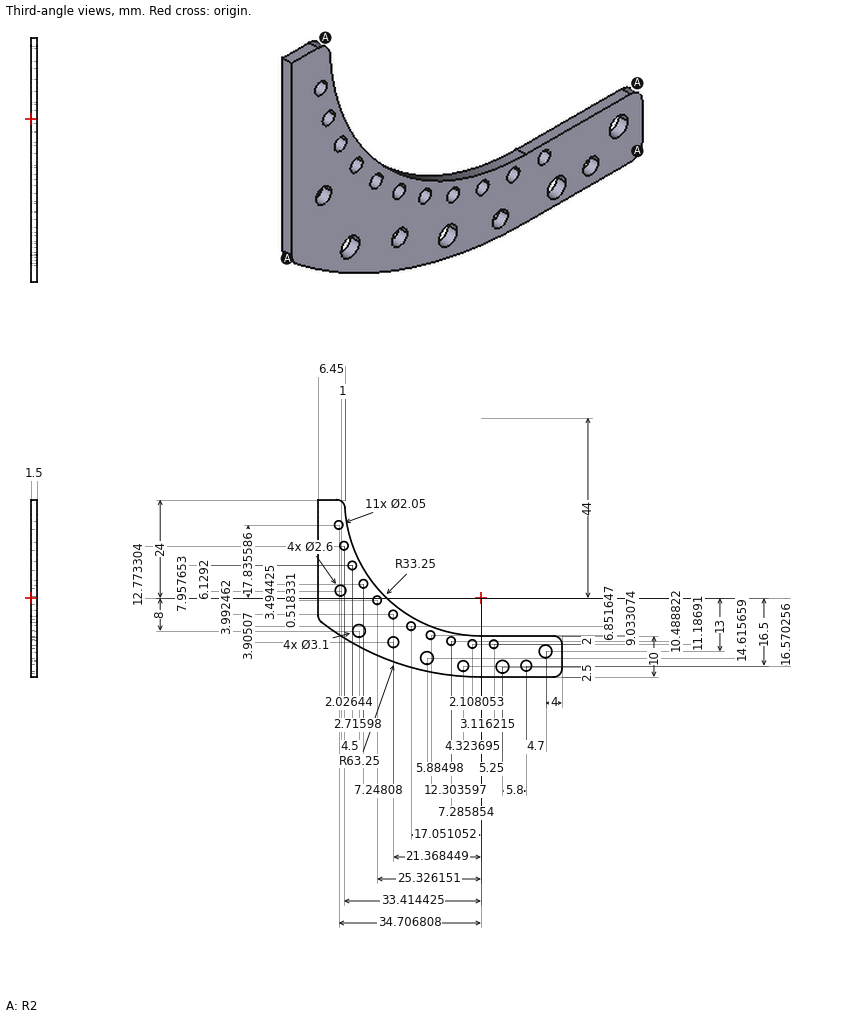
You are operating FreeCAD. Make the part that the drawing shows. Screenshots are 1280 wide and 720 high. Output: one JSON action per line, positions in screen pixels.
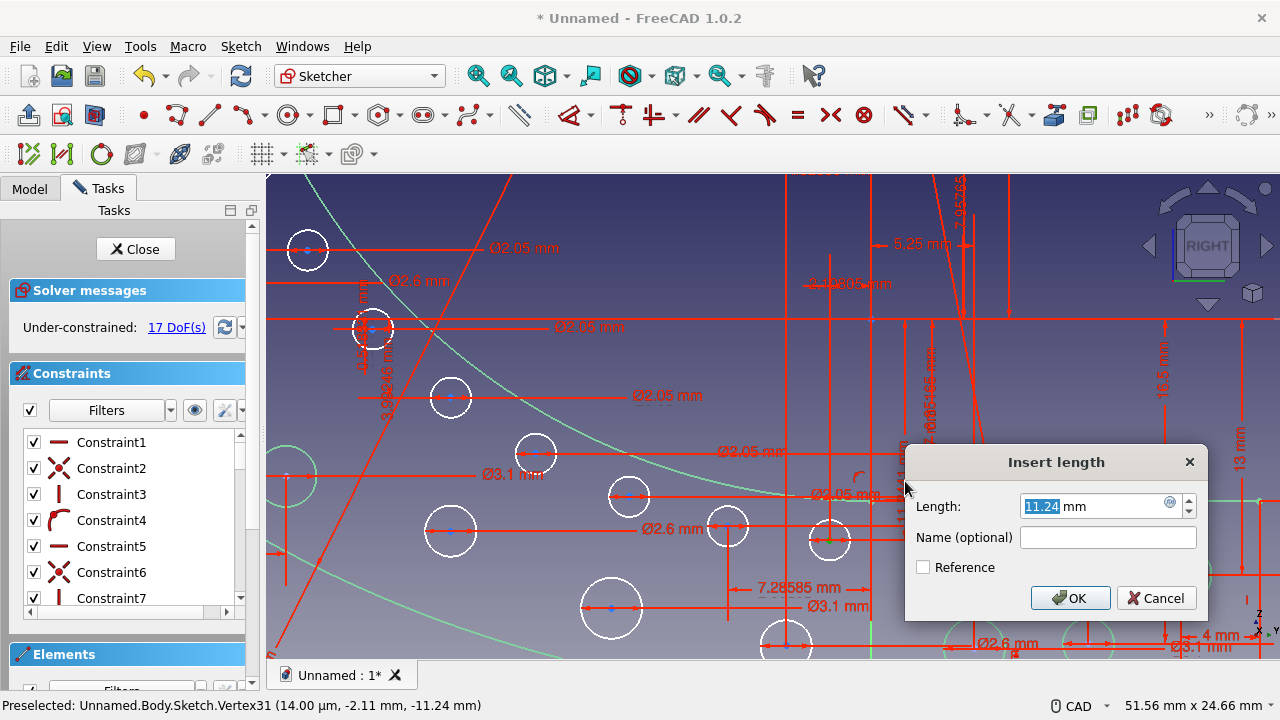
{"action": "type", "text": "11.18691"}
{"action": "key", "text": "Return"}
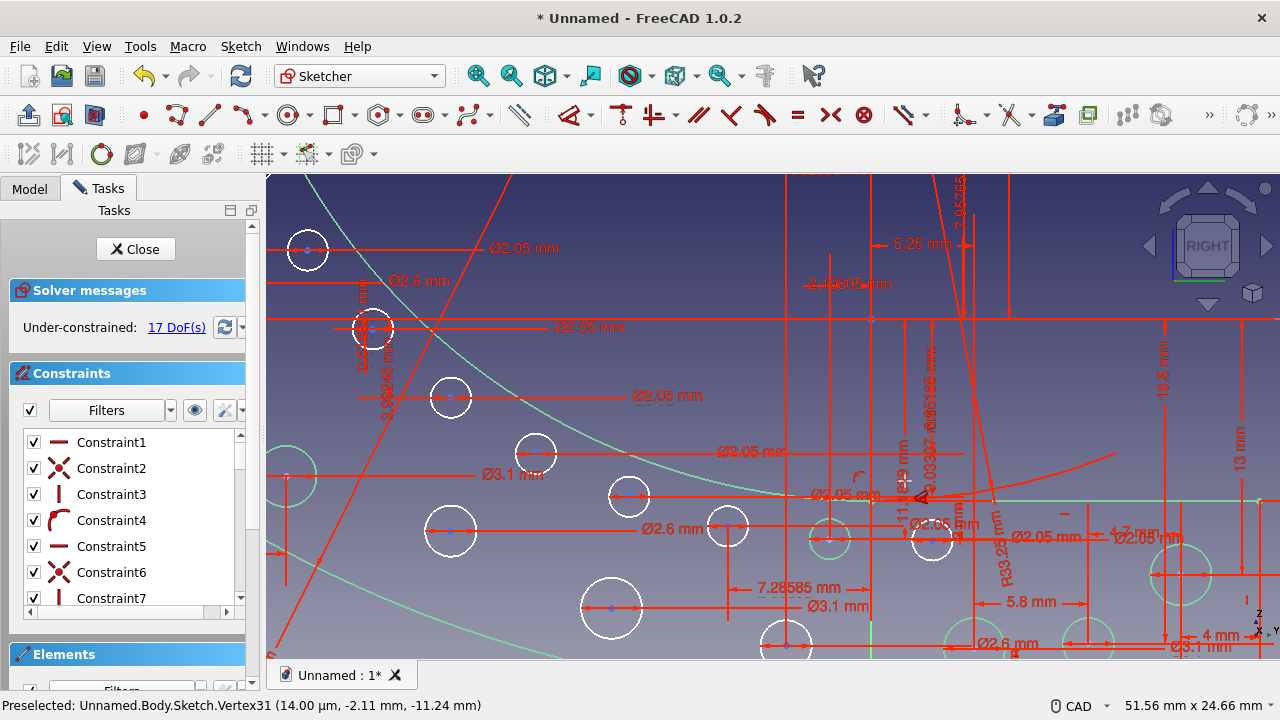
{"action": "left_click", "coordinate": [932, 540]}
{"action": "left_click", "coordinate": [902, 574]}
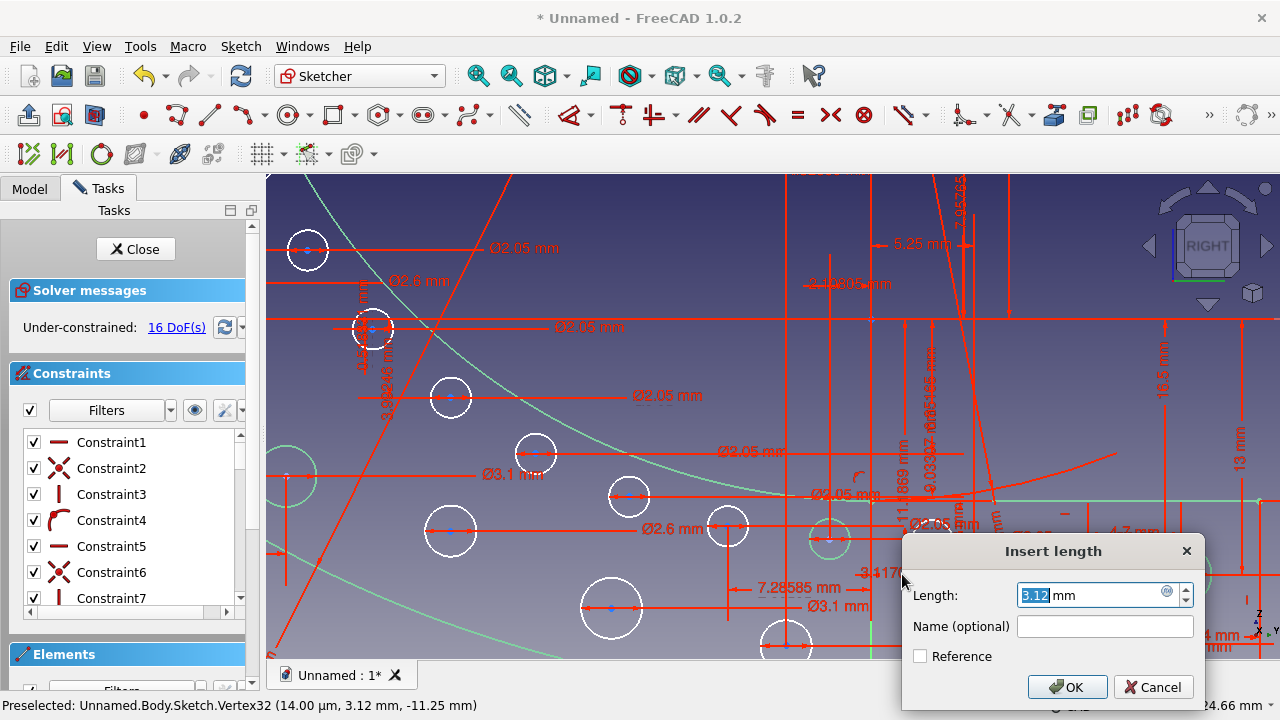
{"action": "type", "text": "3.116215"}
{"action": "key", "text": "Return"}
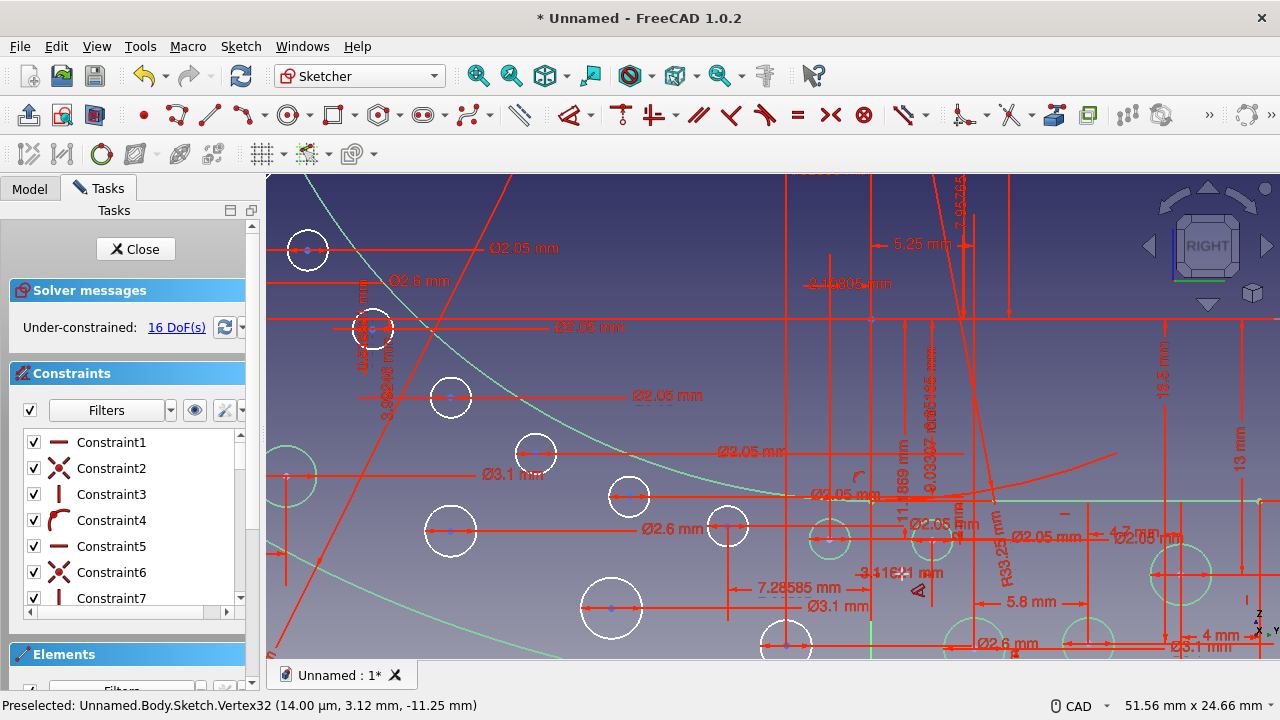
{"action": "scroll", "coordinate": [722, 500], "scroll_direction": "down", "scroll_amount": 5}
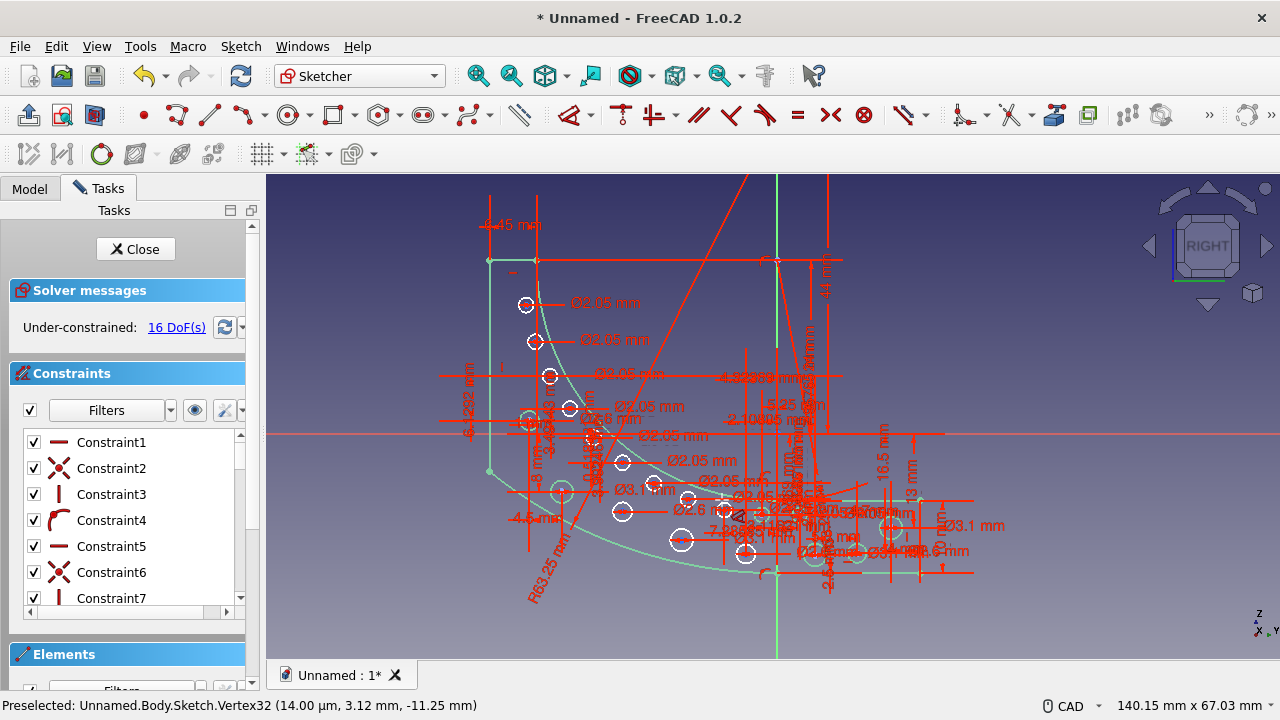
{"action": "scroll", "coordinate": [535, 342], "scroll_direction": "up", "scroll_amount": 5}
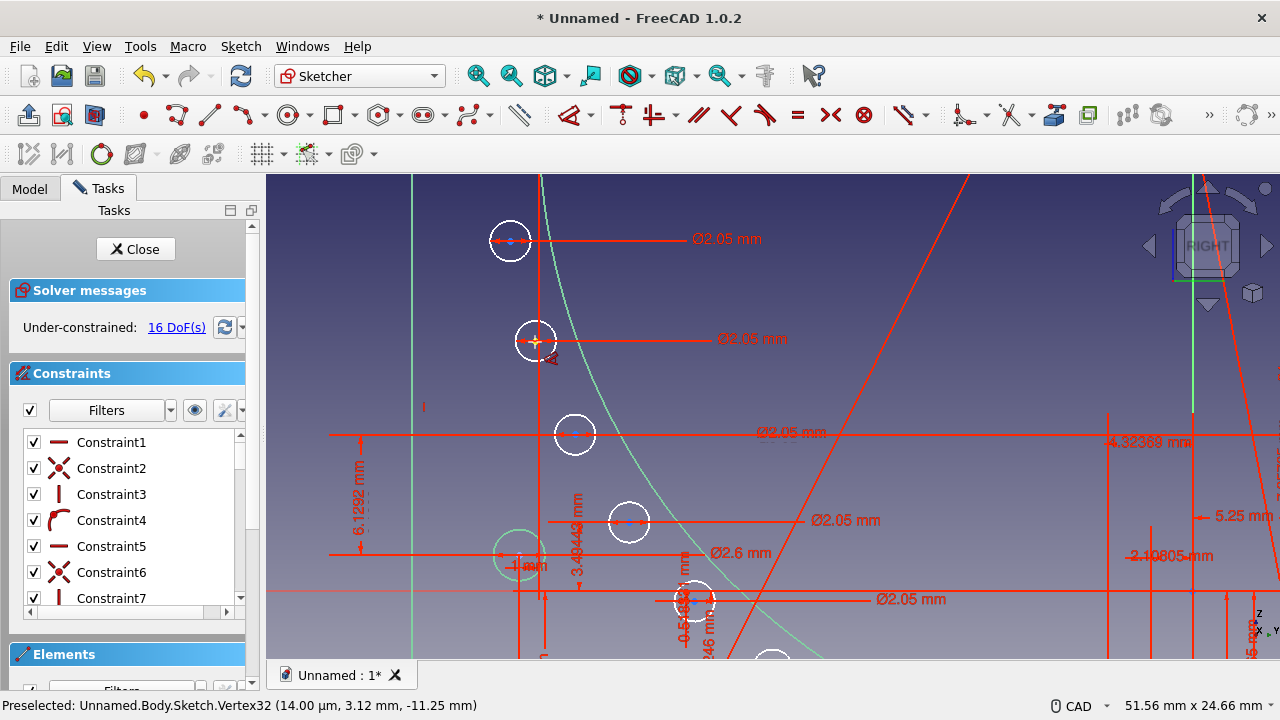
{"action": "left_click", "coordinate": [536, 341]}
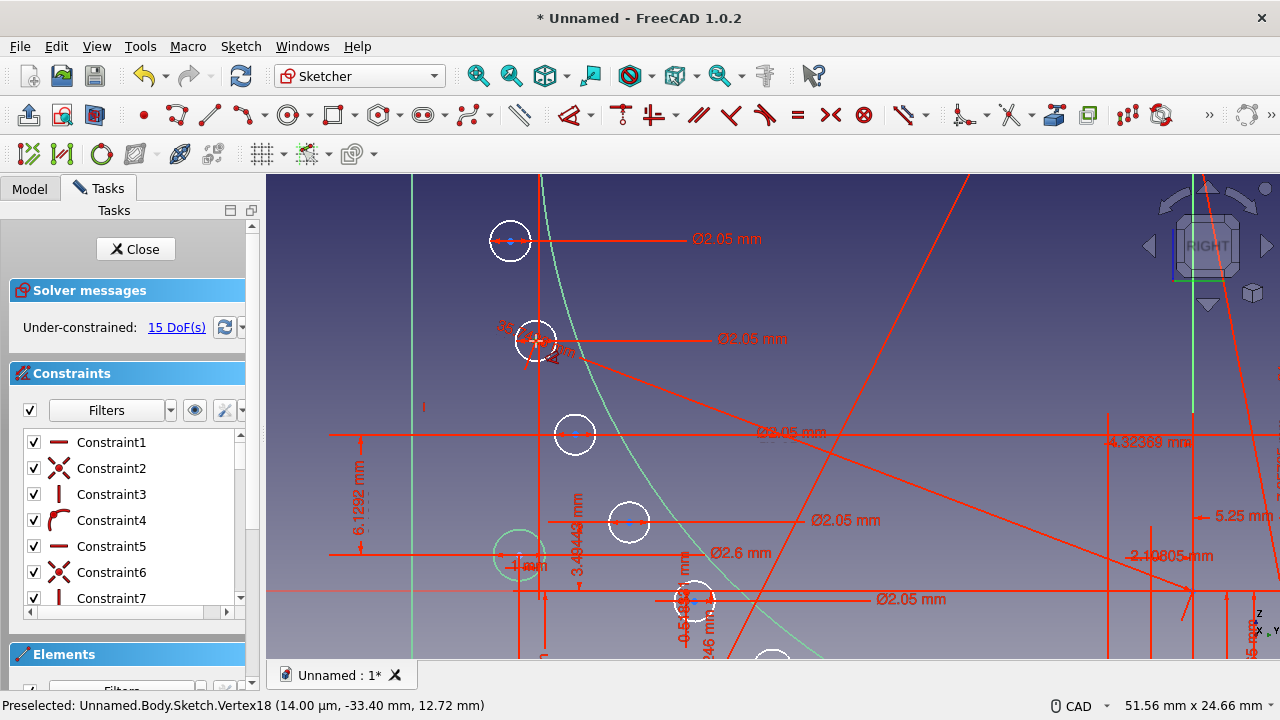
{"action": "left_click", "coordinate": [575, 435]}
{"action": "left_click", "coordinate": [546, 307]}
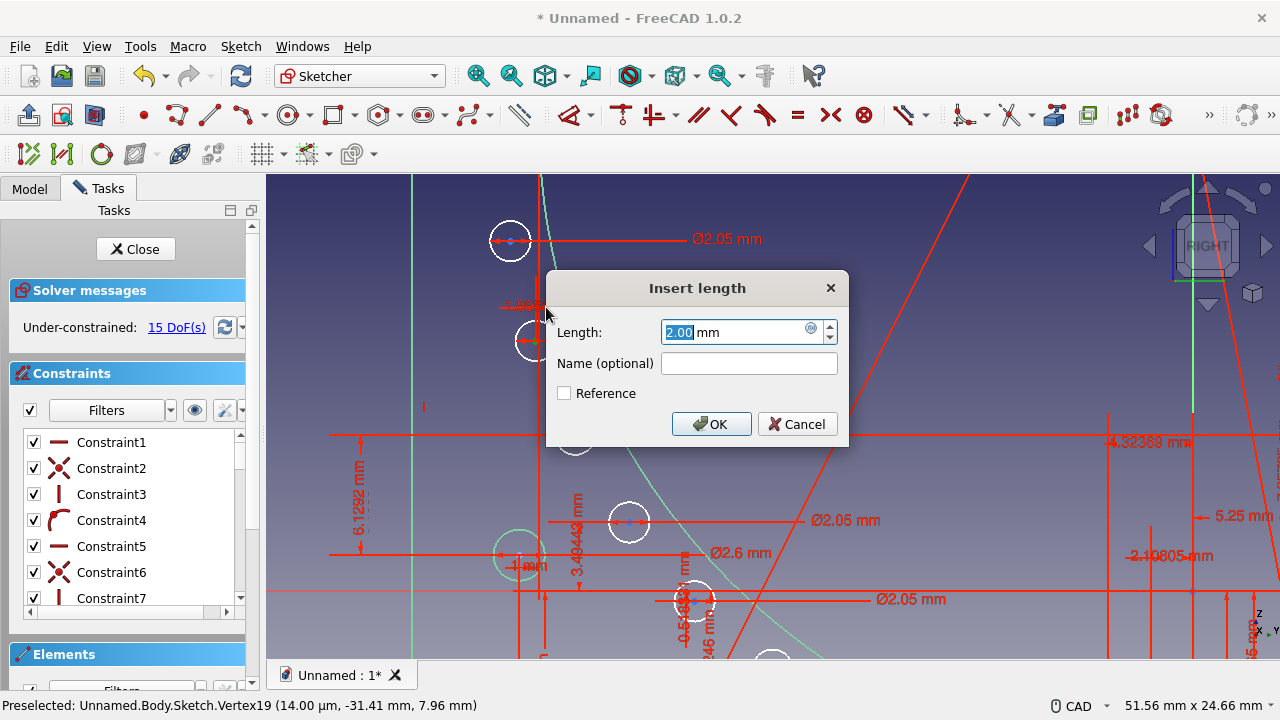
{"action": "type", "text": "2.02644"}
{"action": "key", "text": "Return"}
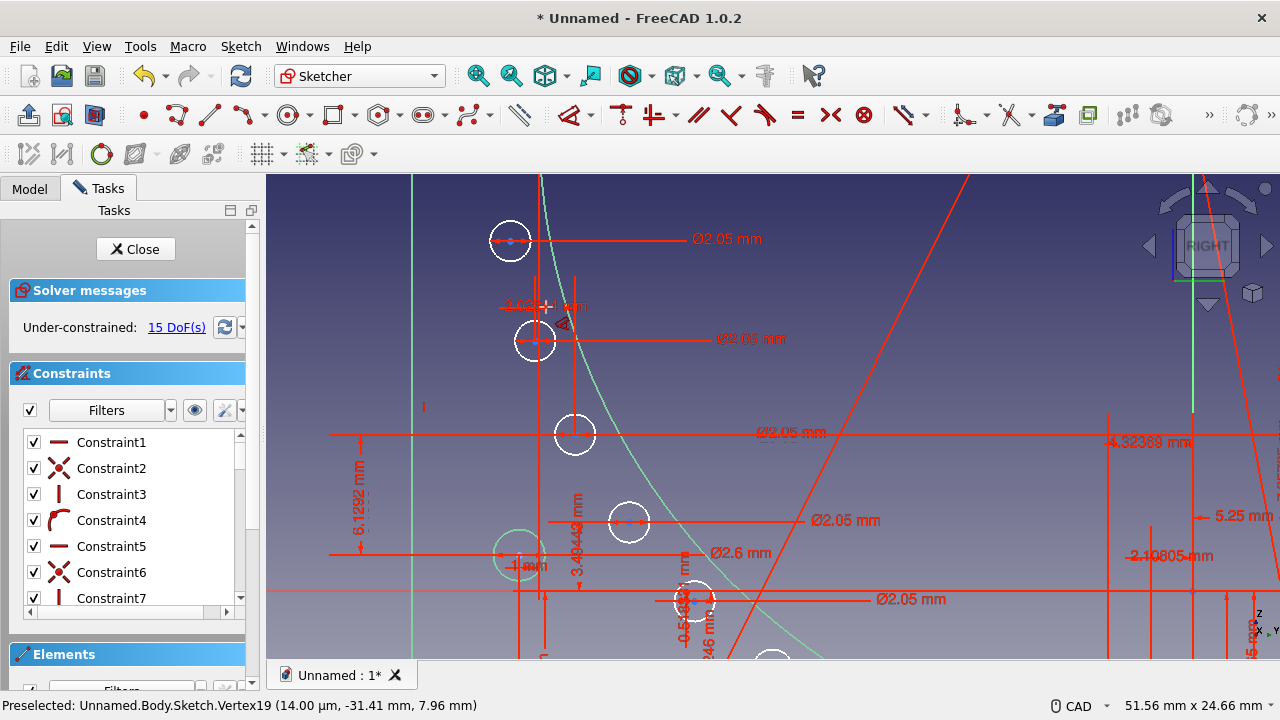
{"action": "left_click", "coordinate": [575, 435]}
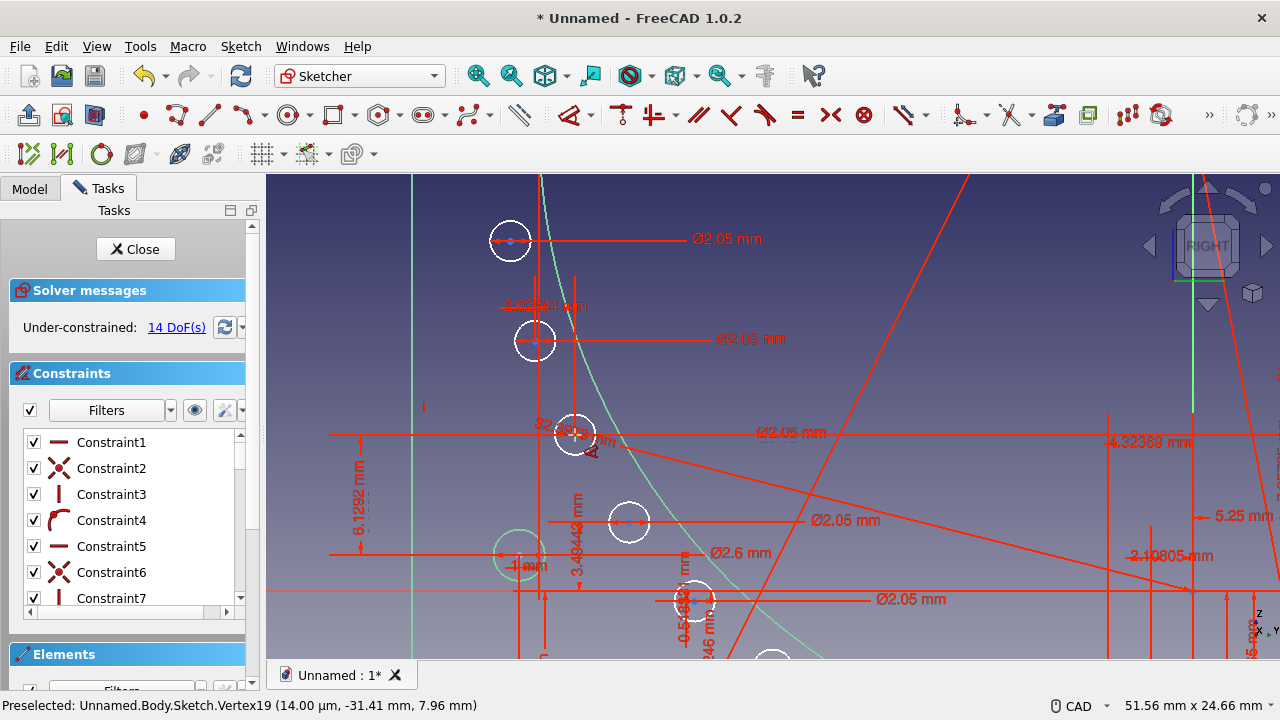
{"action": "left_click", "coordinate": [629, 522]}
{"action": "left_click", "coordinate": [583, 401]}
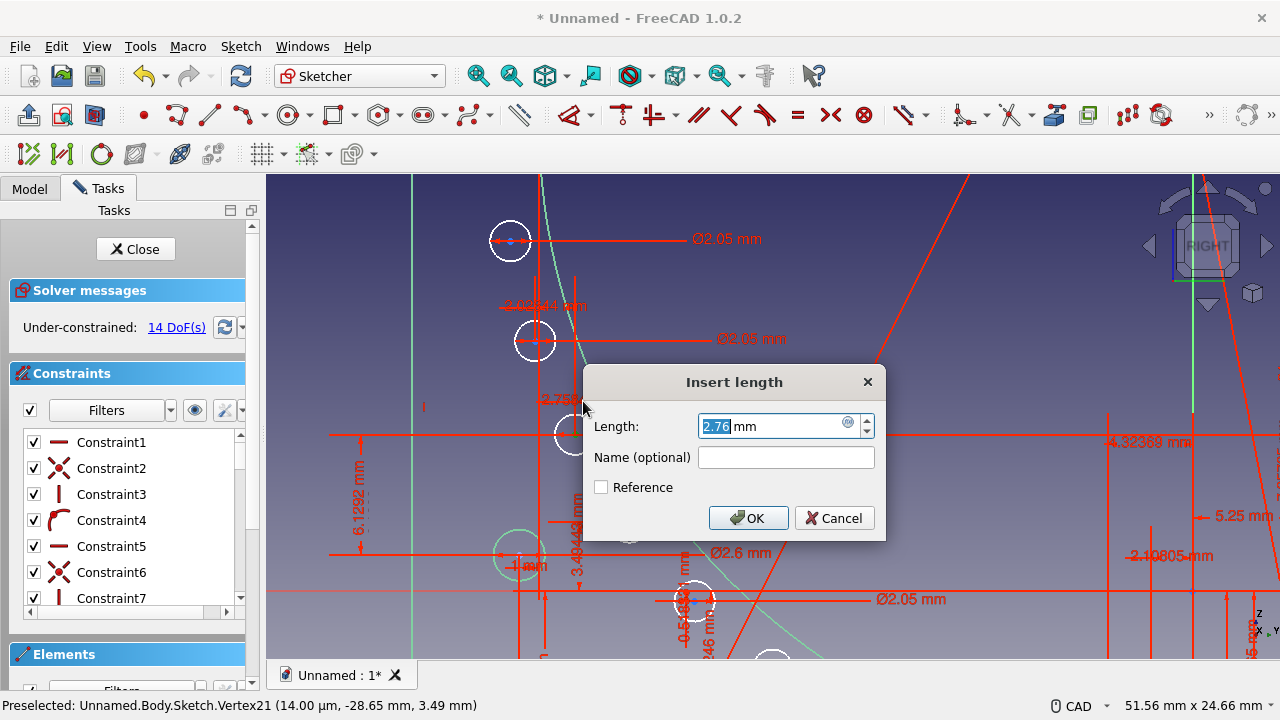
{"action": "type", "text": "2.71598"}
{"action": "key", "text": "Return"}